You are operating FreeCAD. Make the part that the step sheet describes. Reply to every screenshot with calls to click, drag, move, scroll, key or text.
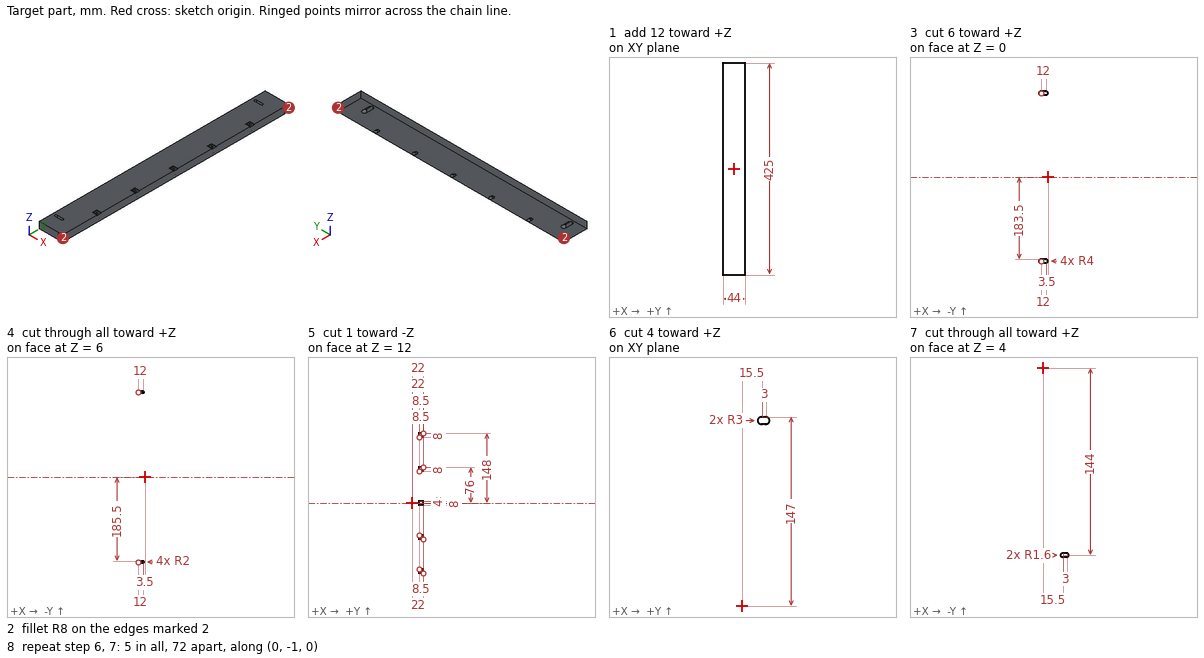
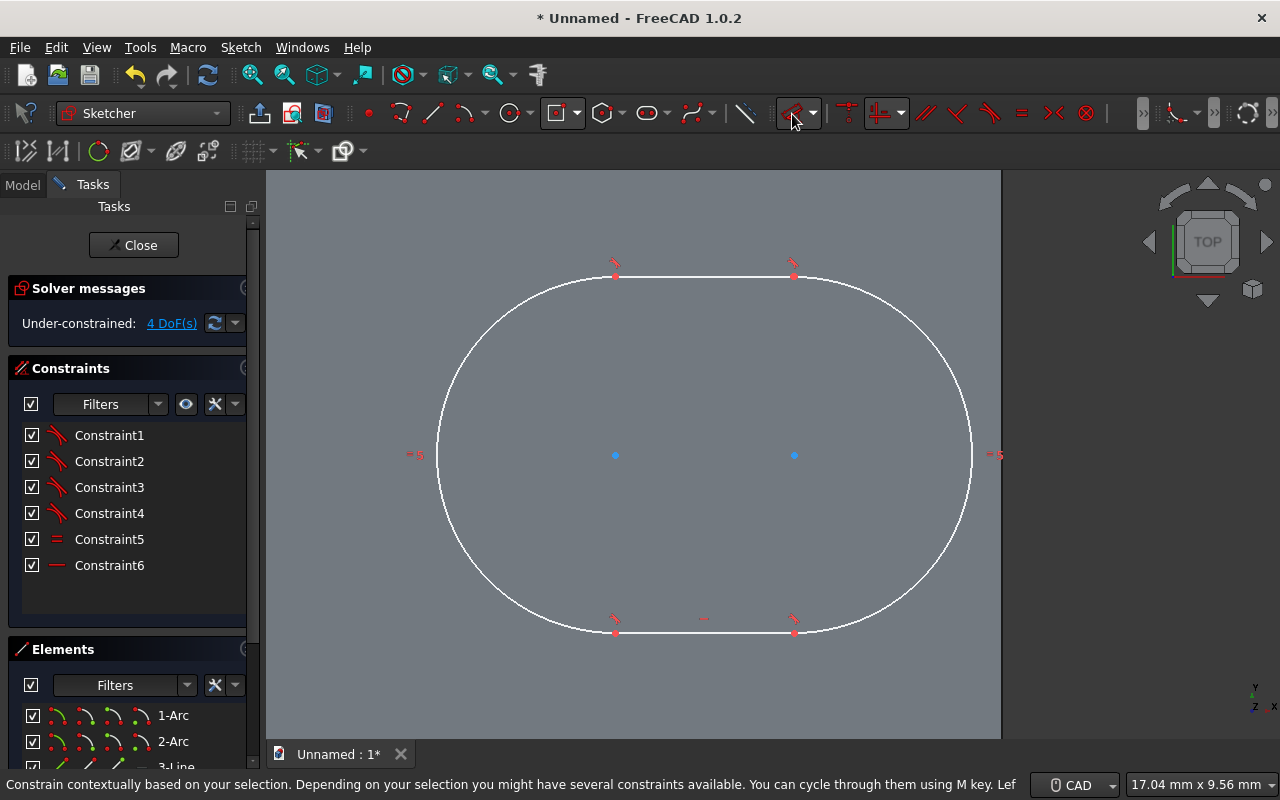
click(471, 350)
click(445, 331)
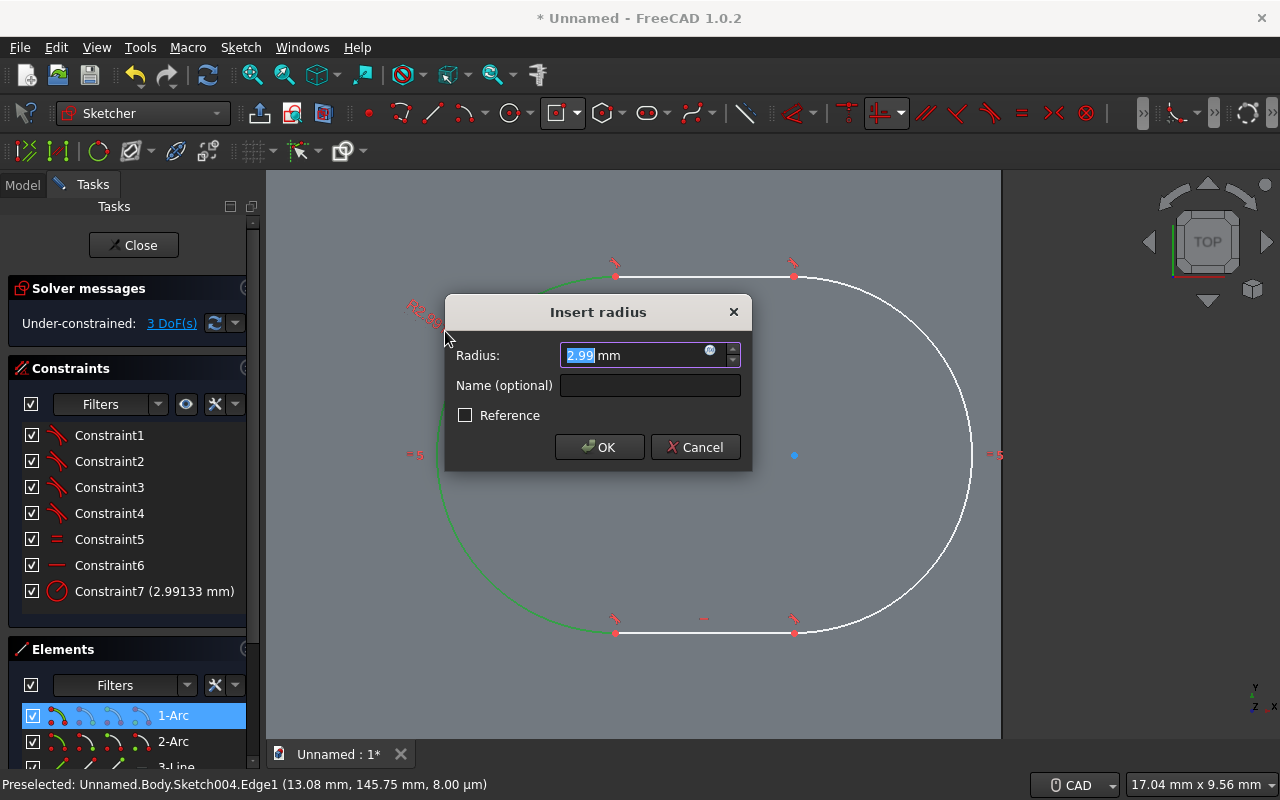
text(3)
key(Return)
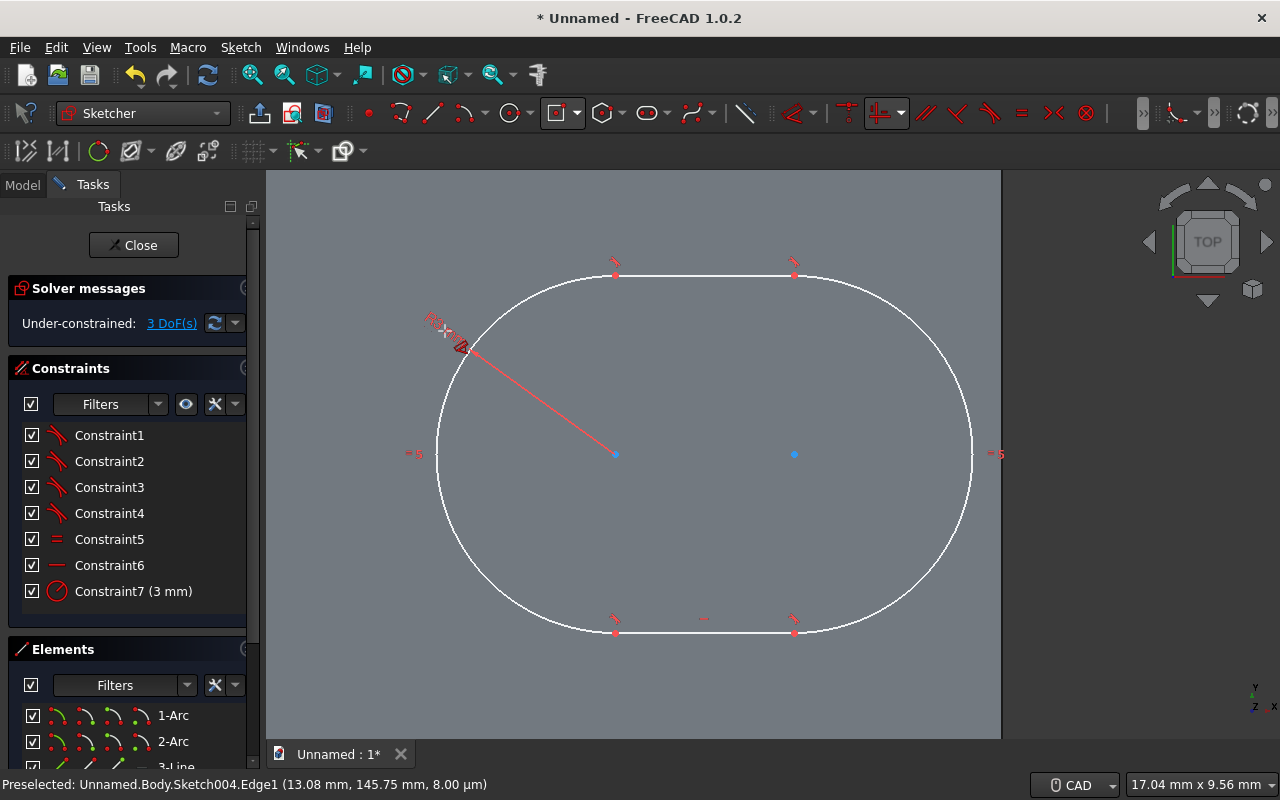
click(669, 276)
click(704, 242)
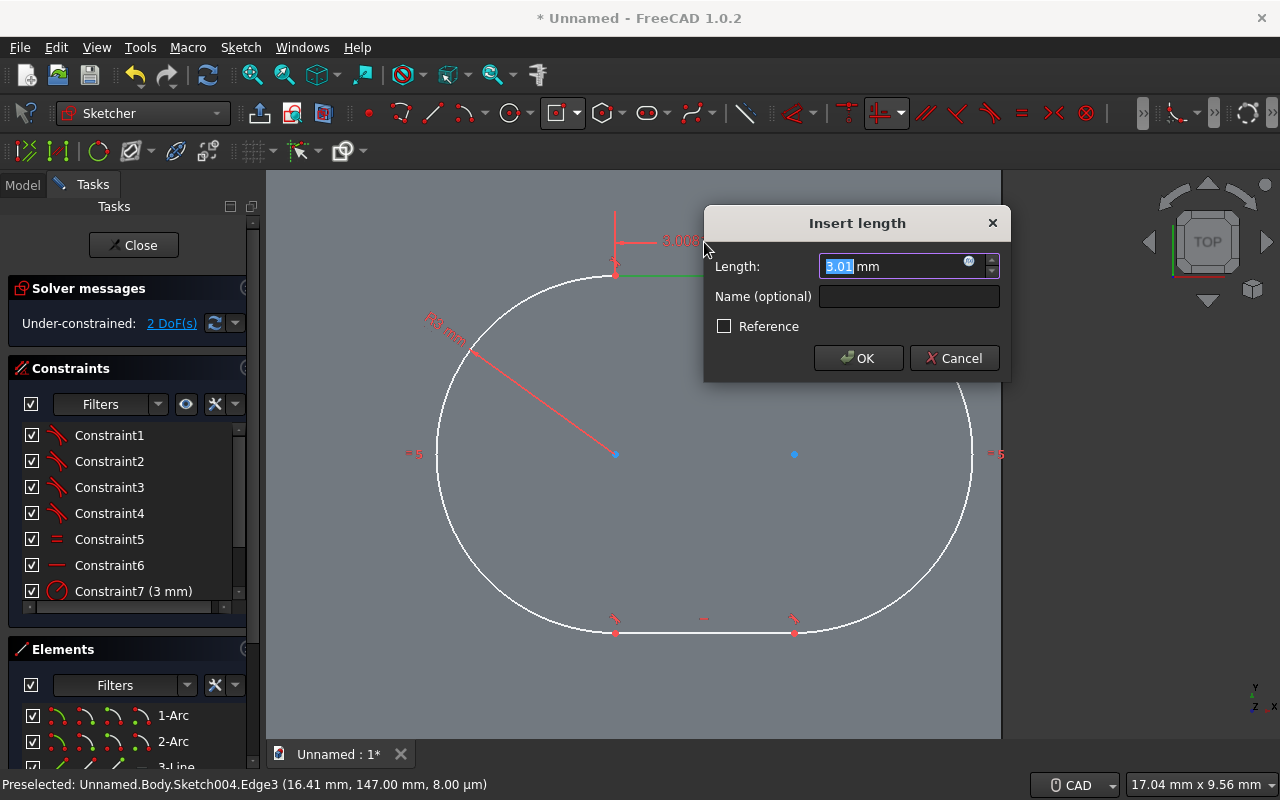
text(3)
key(Return)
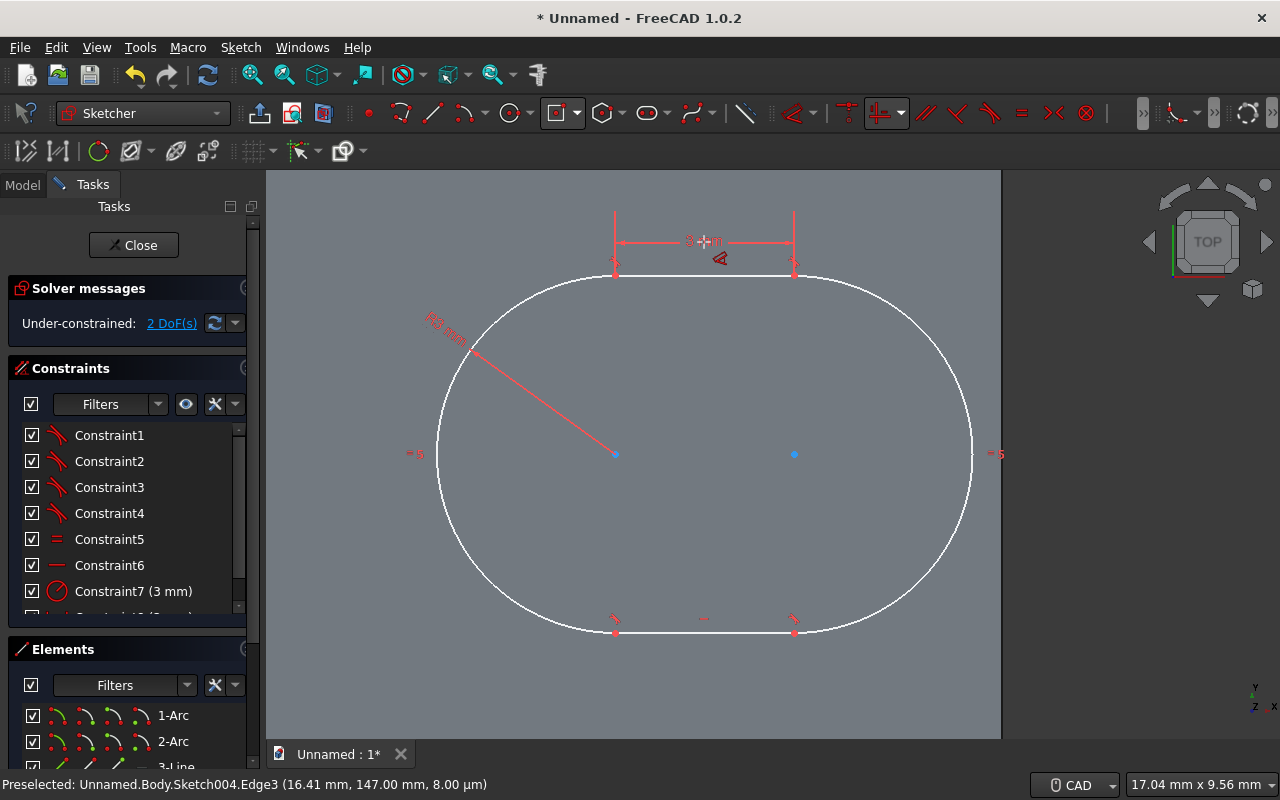
click(615, 276)
click(649, 493)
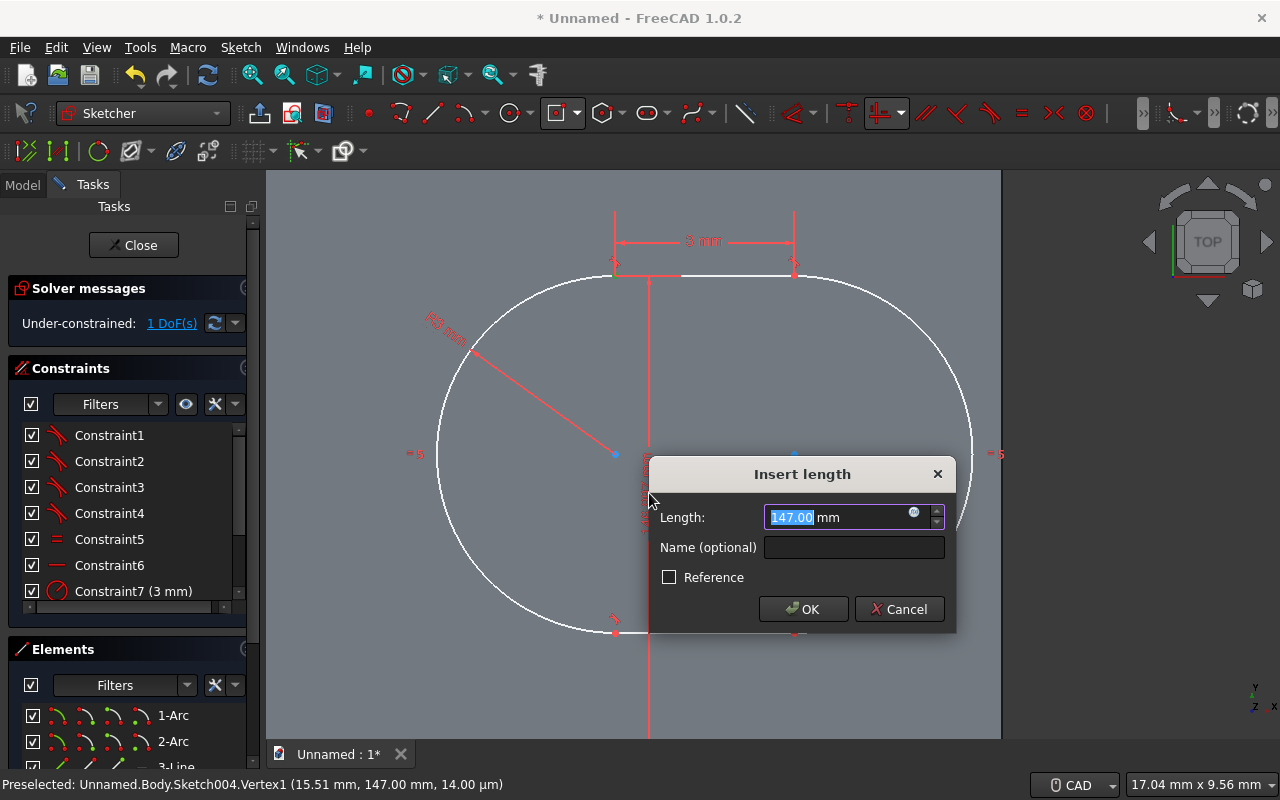
text(147)
key(Return)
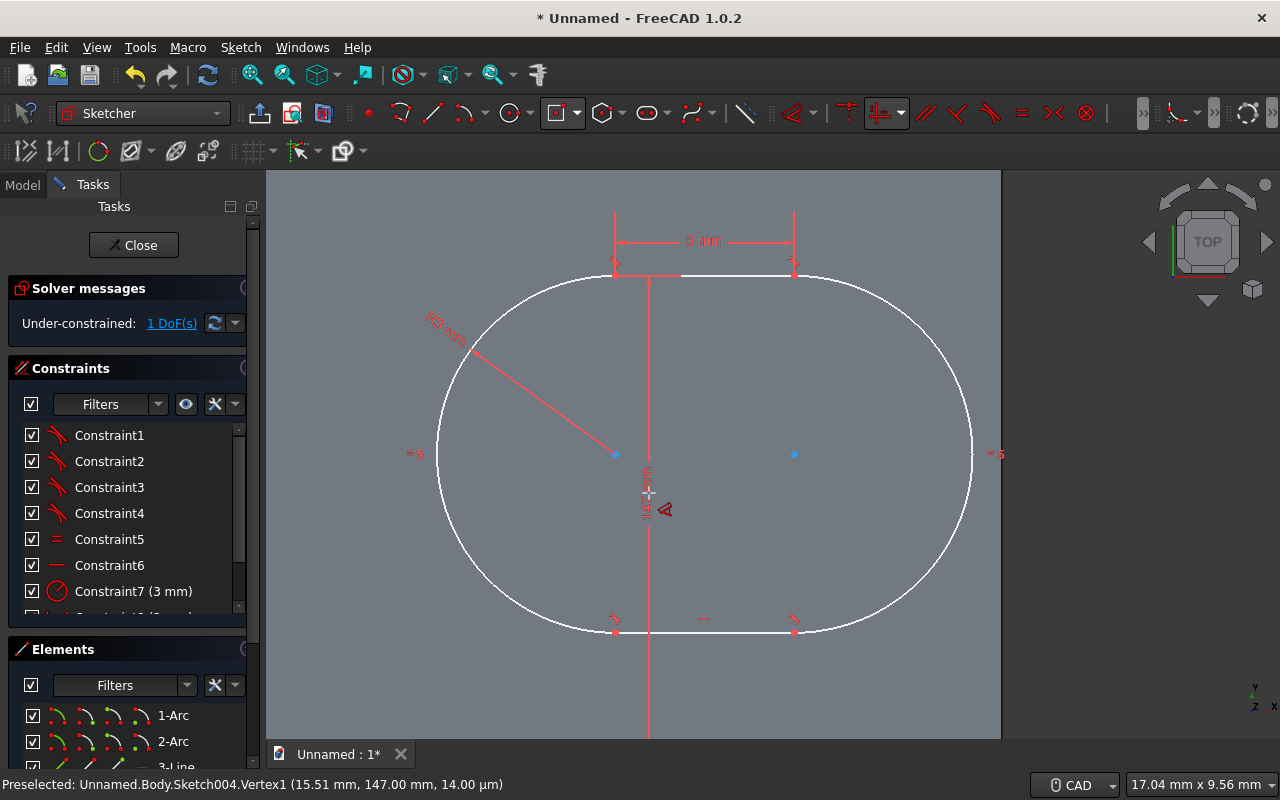
click(615, 276)
click(455, 242)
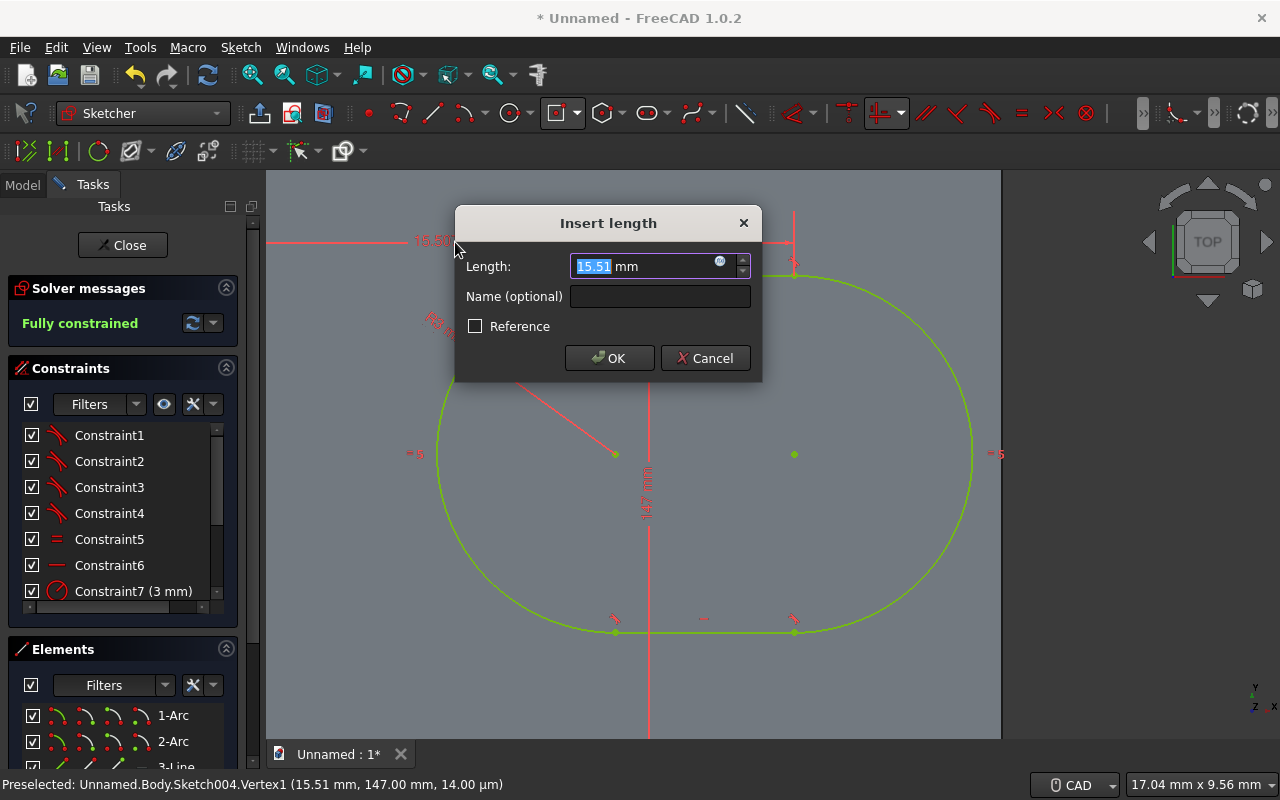
text(15.5)
key(Return)
key(Escape)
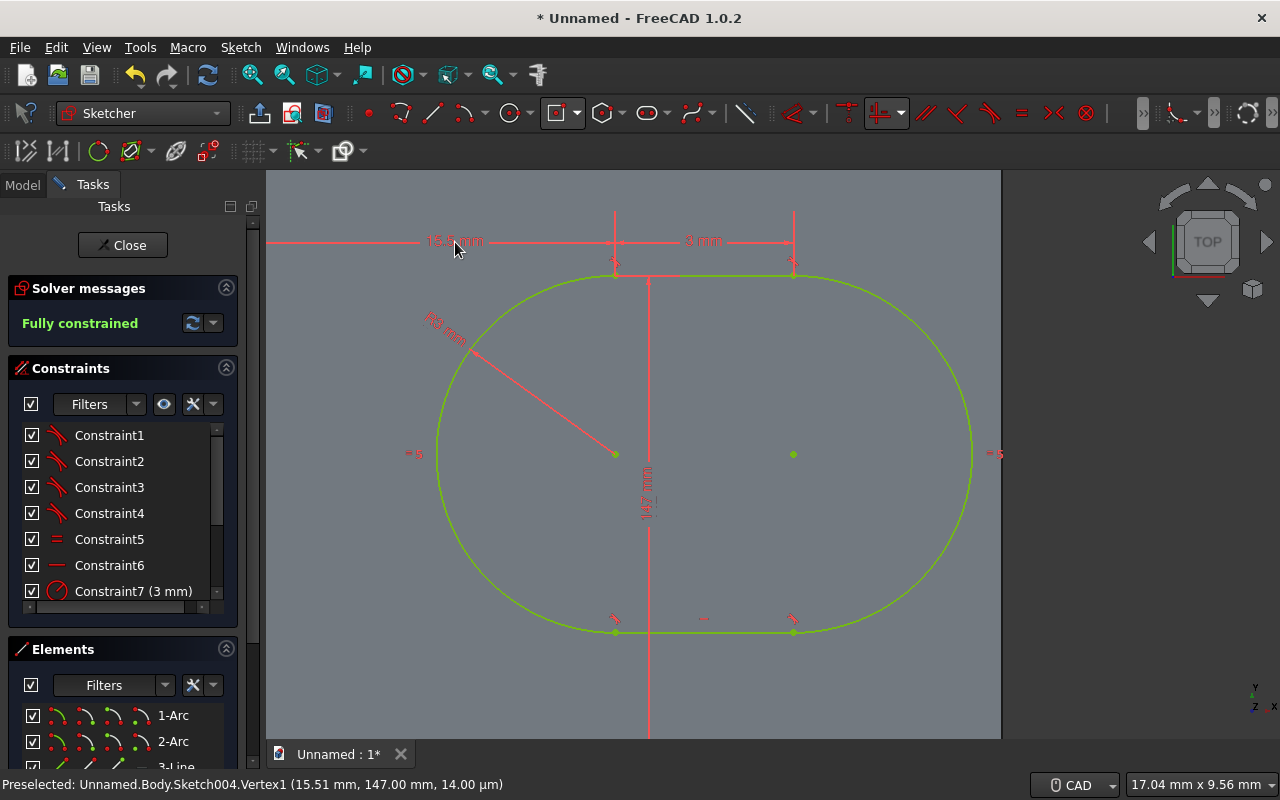
click(123, 245)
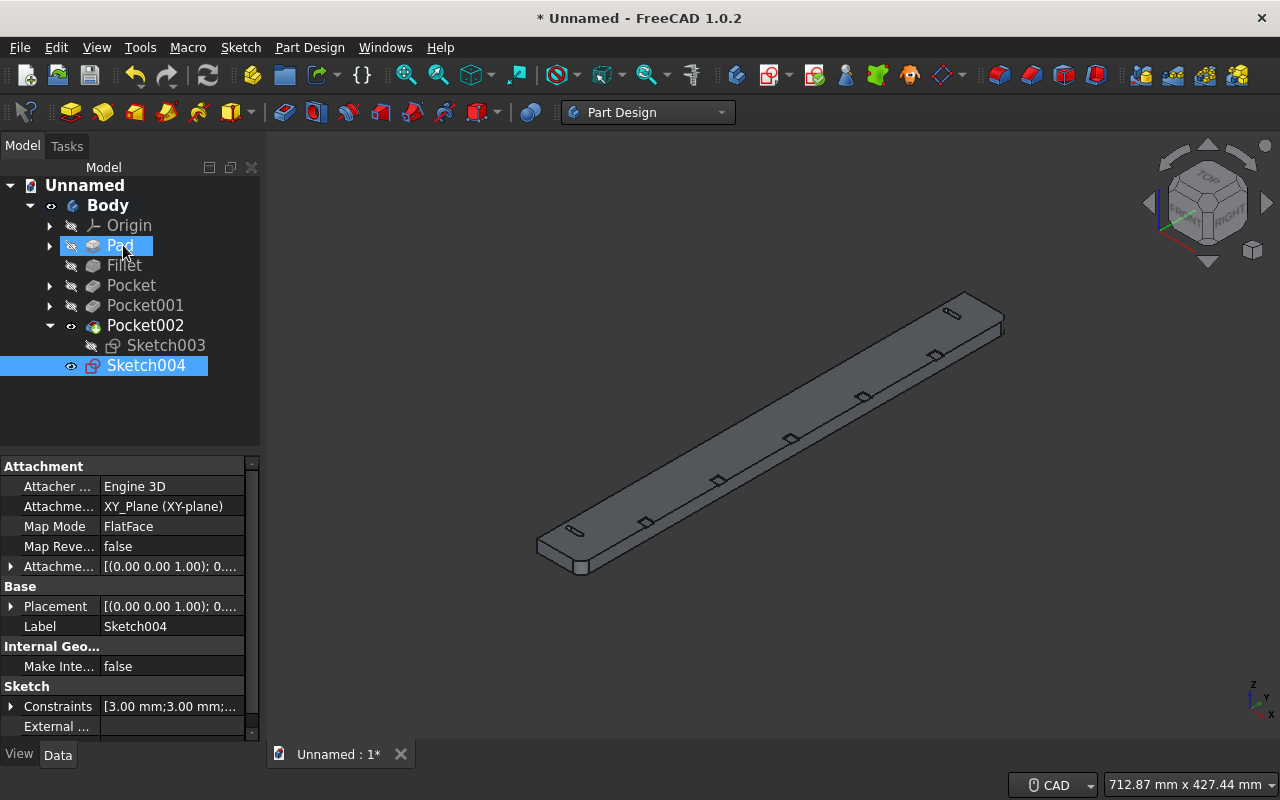
click(286, 112)